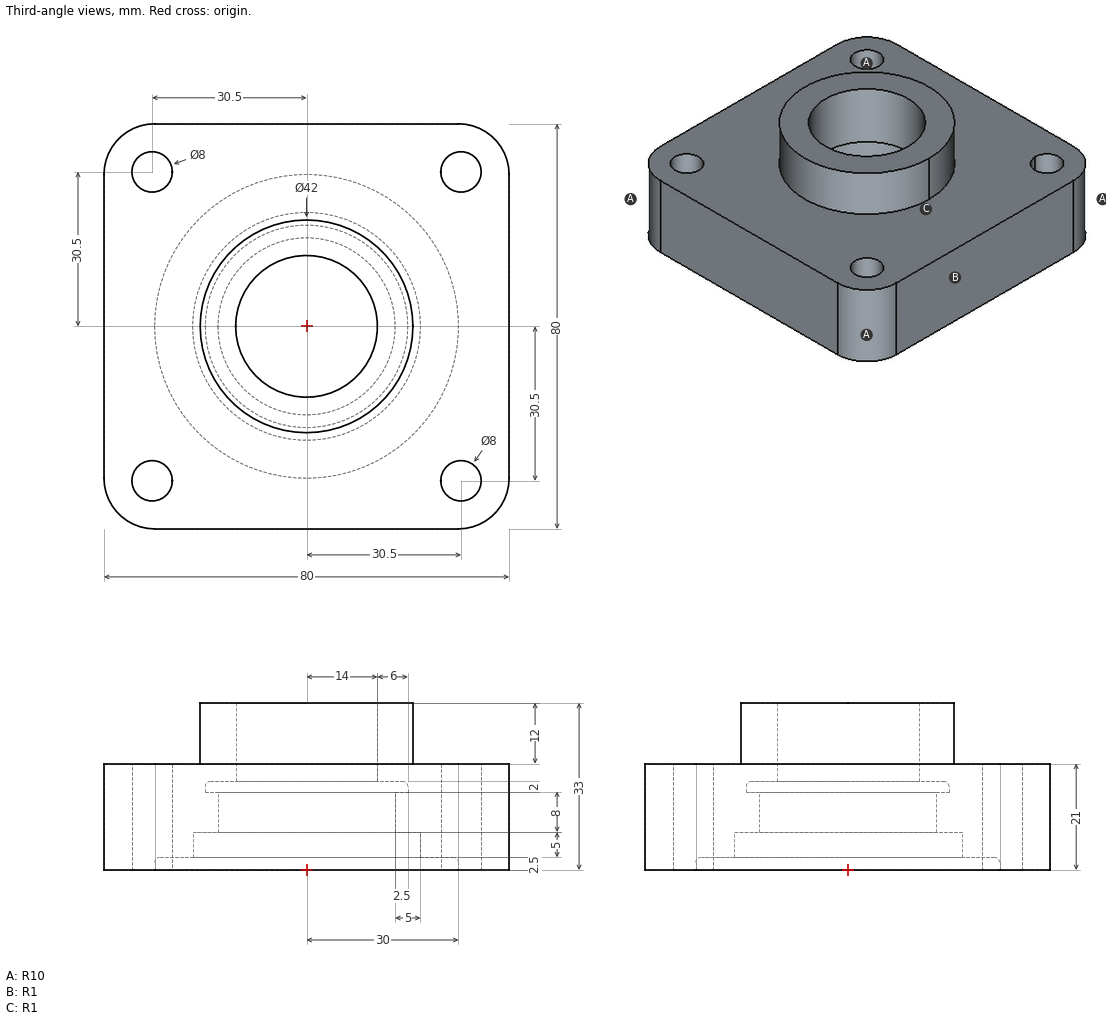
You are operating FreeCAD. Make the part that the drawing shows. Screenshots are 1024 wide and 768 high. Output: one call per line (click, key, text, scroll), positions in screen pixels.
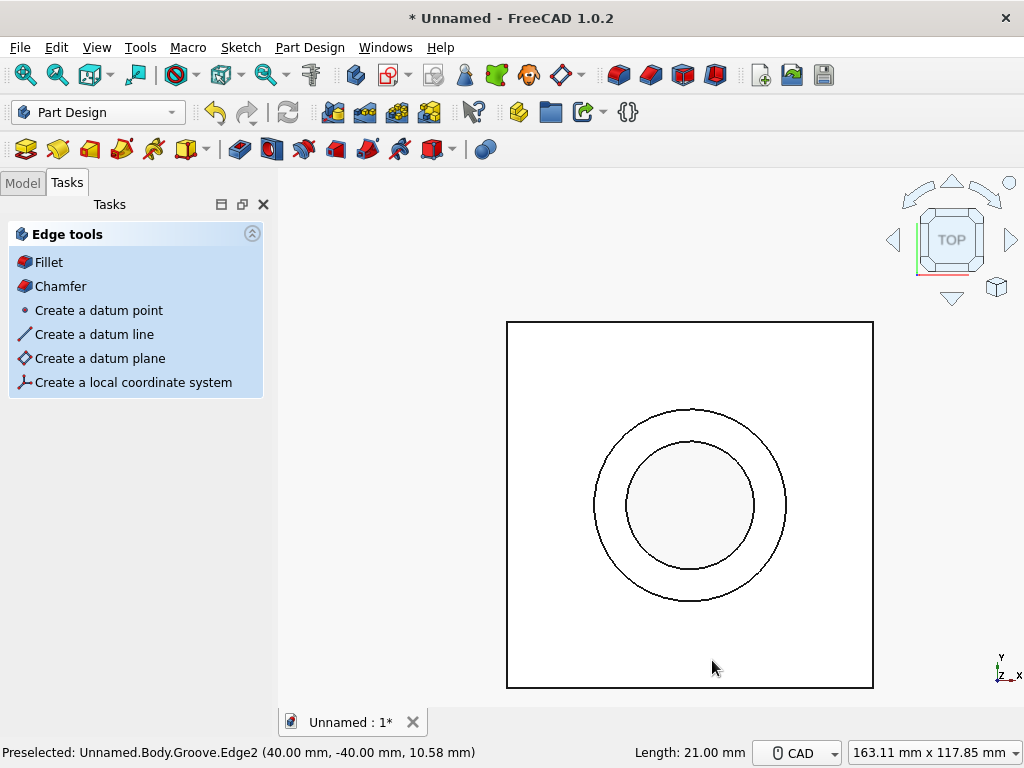
key(1)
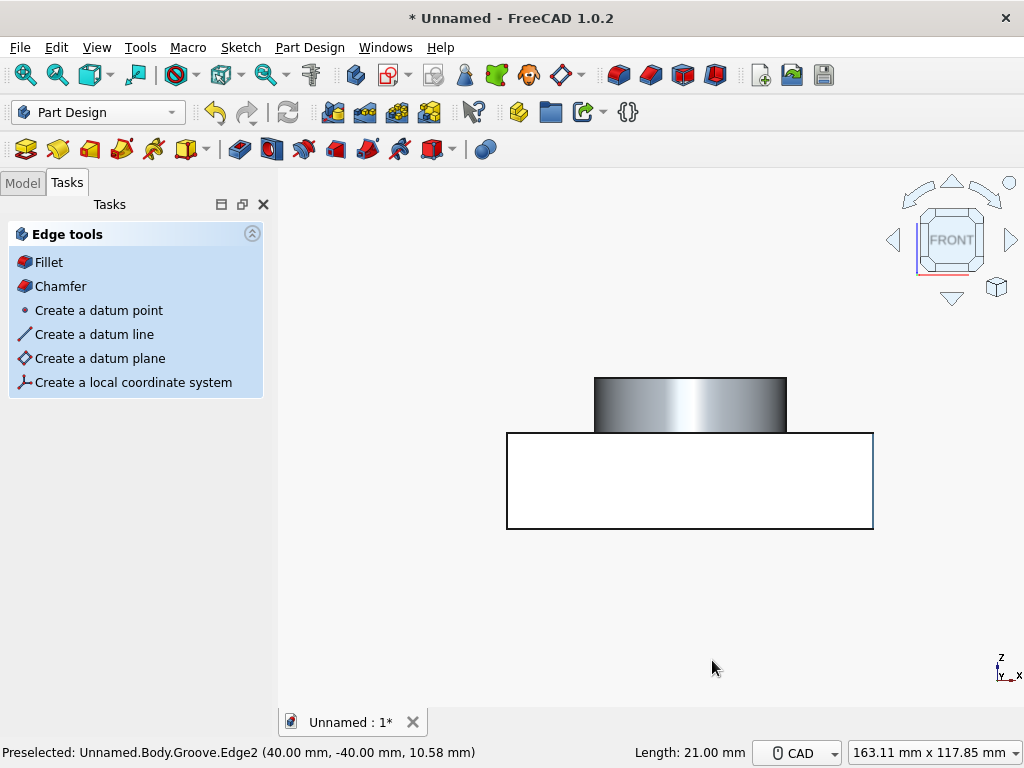
click(507, 480, ctrl)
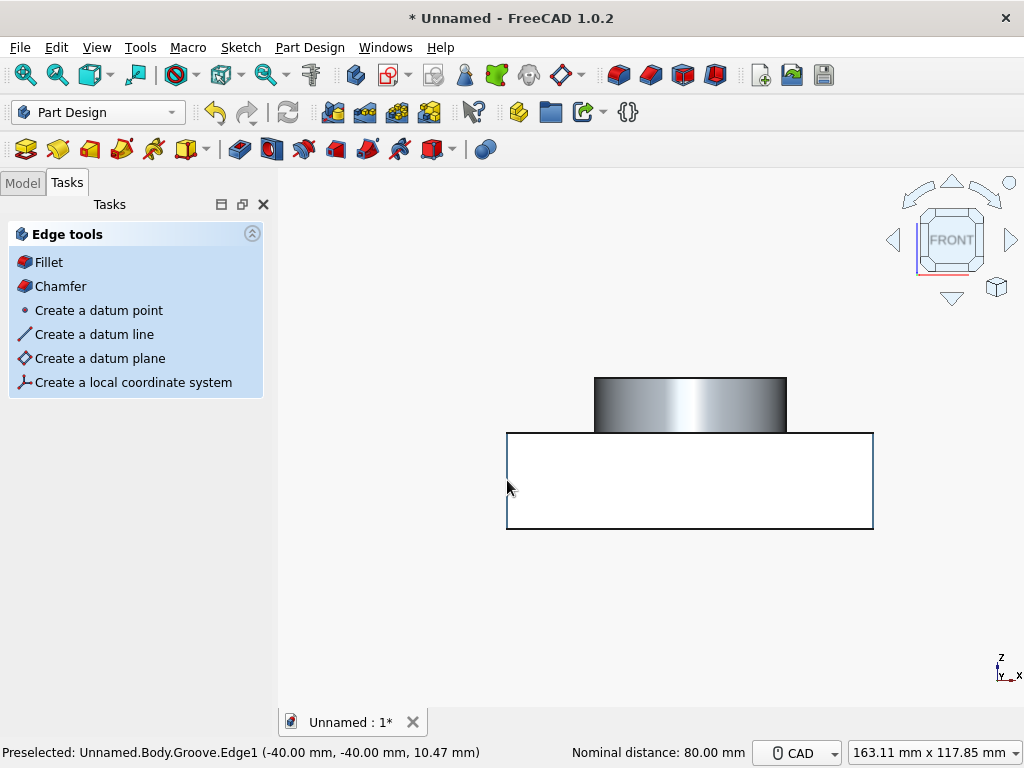
key(3)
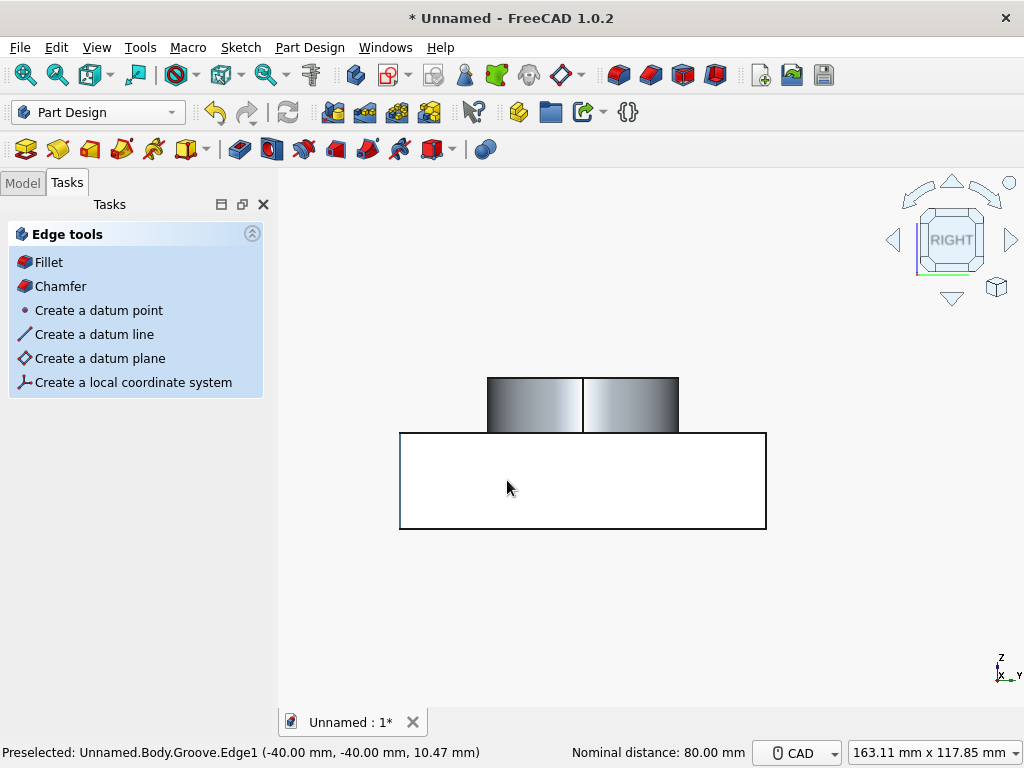
click(766, 480, ctrl)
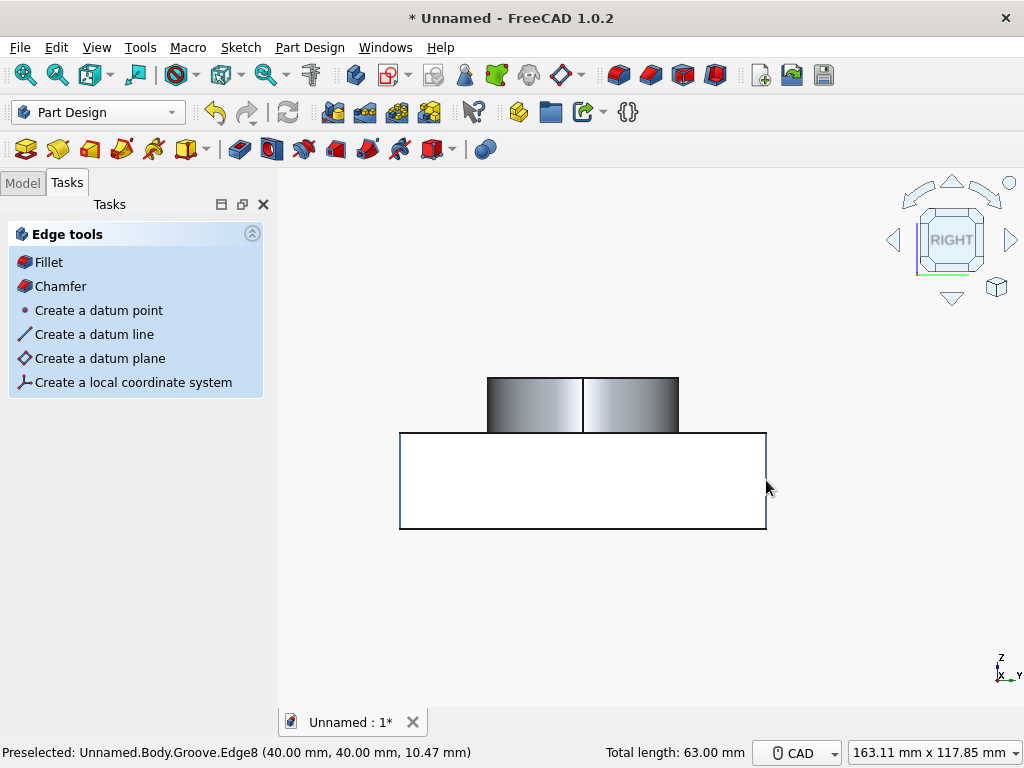
key(5)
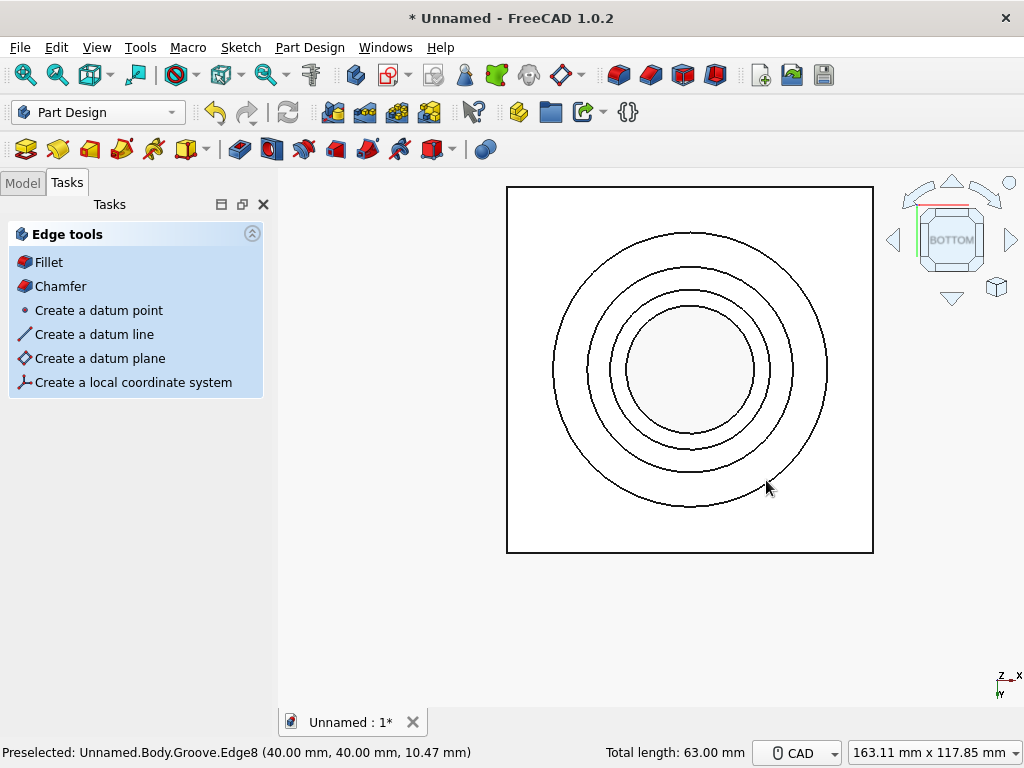
key(4)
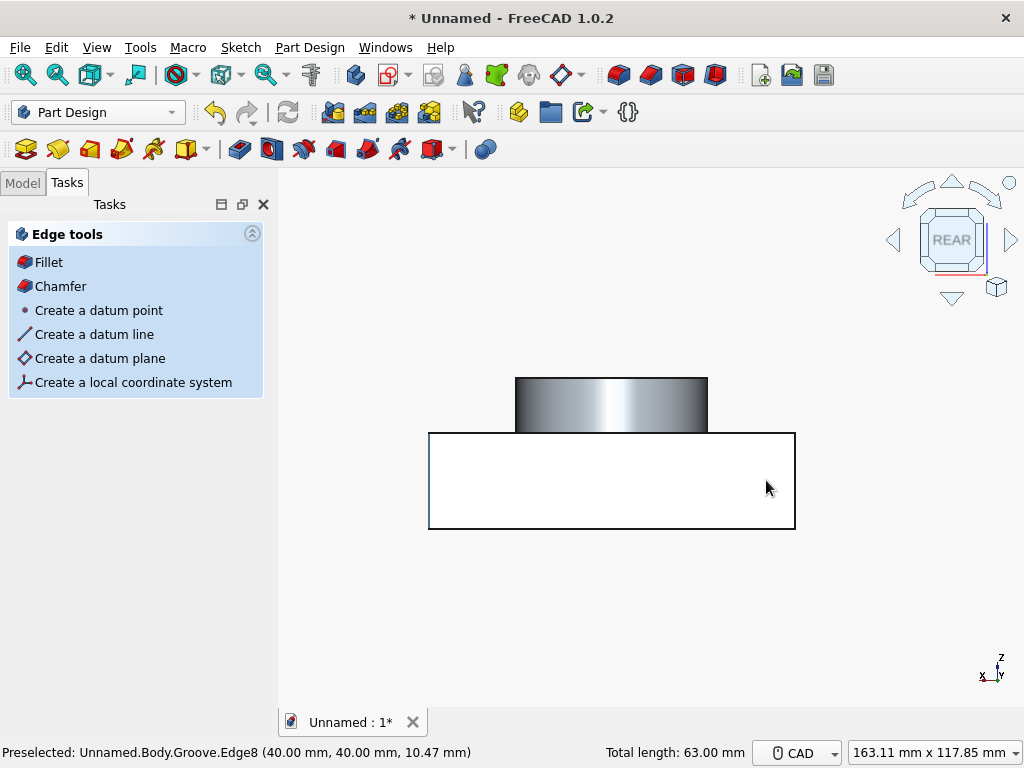
click(795, 480, ctrl)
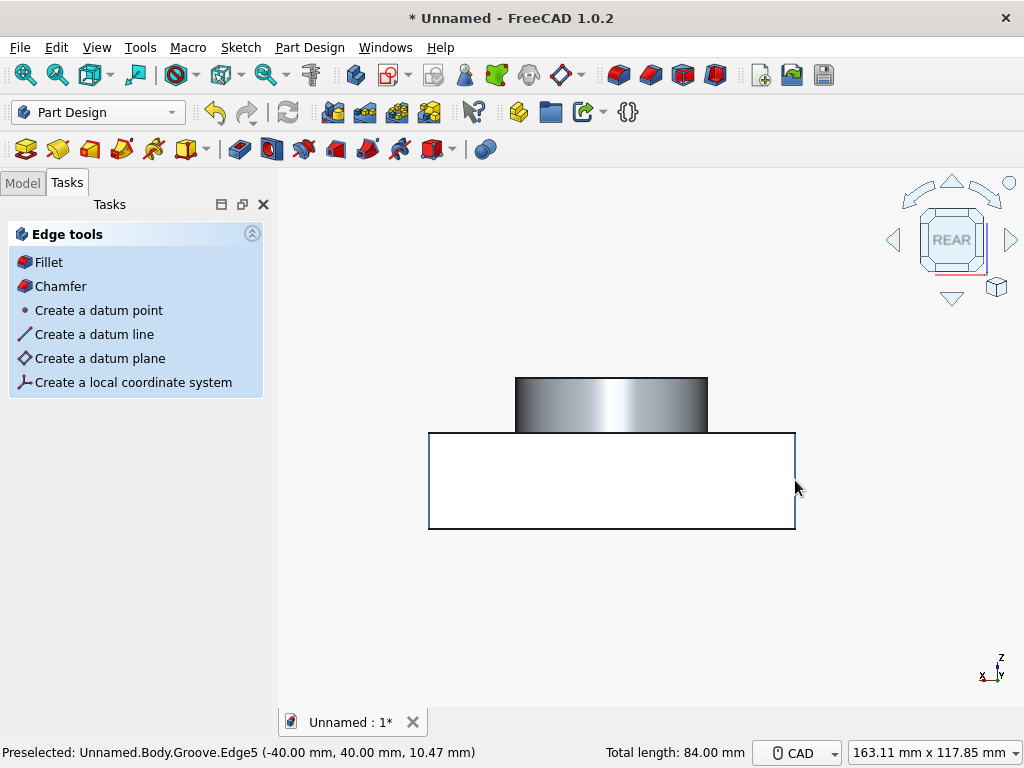
click(620, 76)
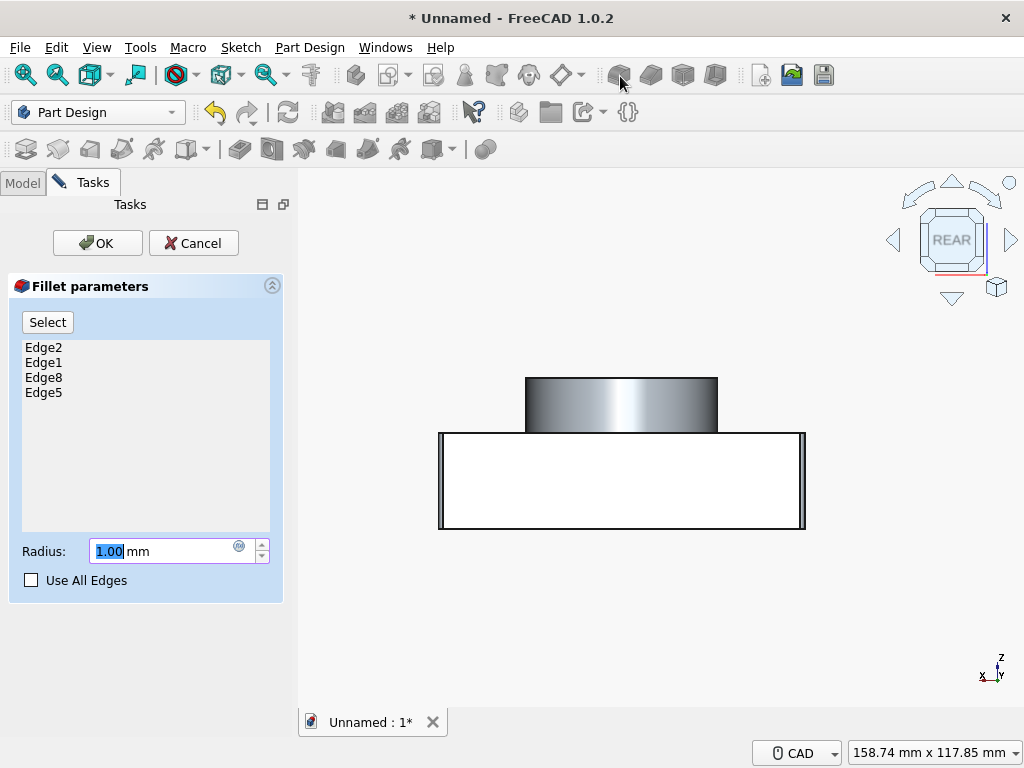
text(10)
key(Tab)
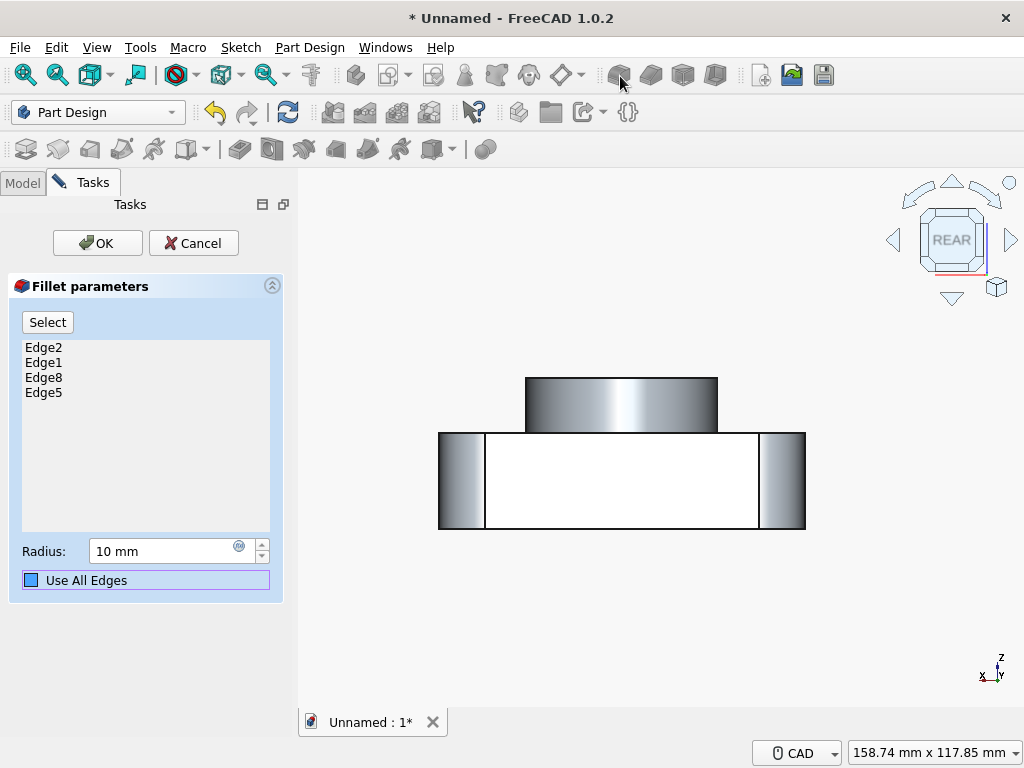
click(98, 243)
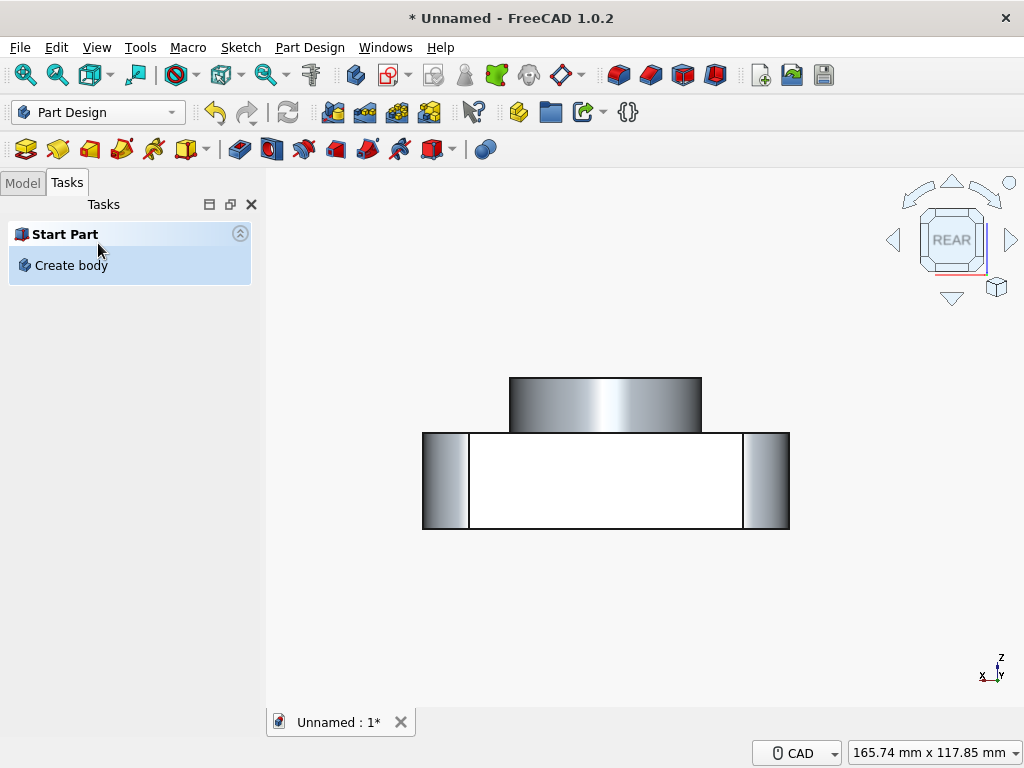
key(0)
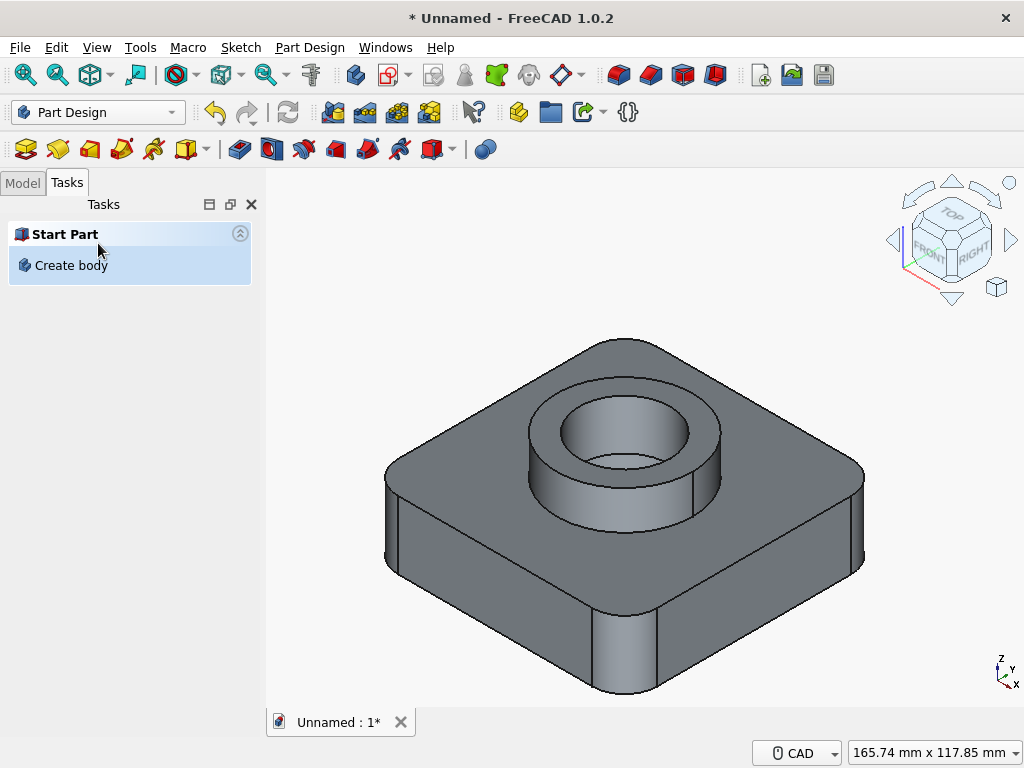
click(625, 562)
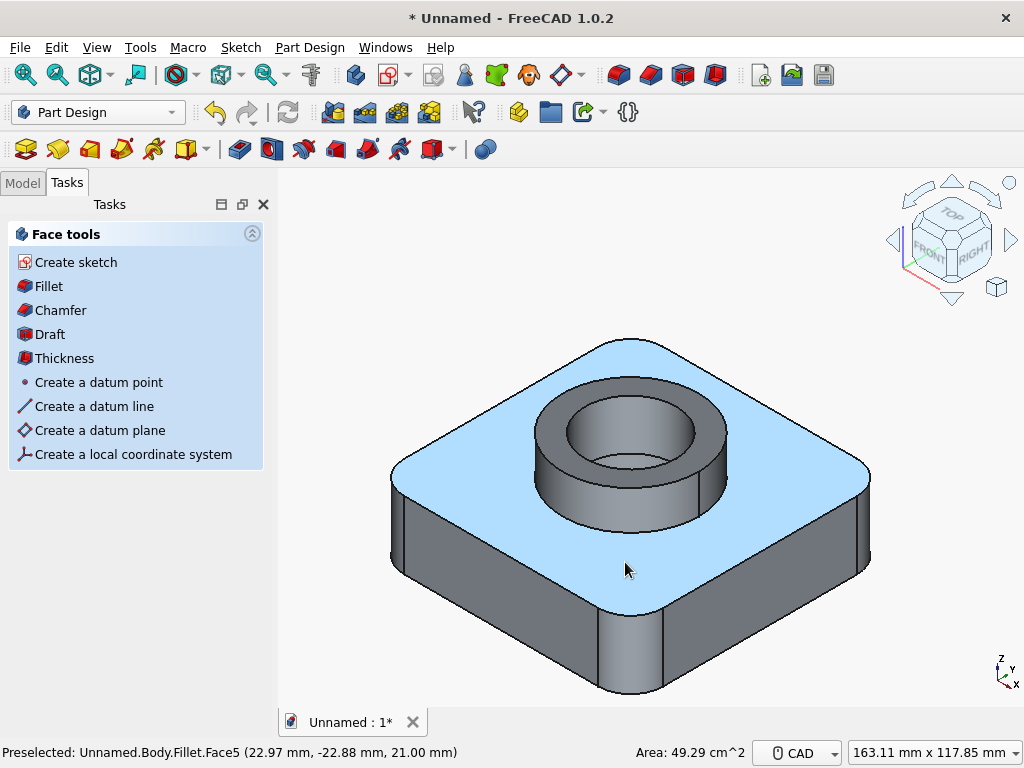
click(388, 76)